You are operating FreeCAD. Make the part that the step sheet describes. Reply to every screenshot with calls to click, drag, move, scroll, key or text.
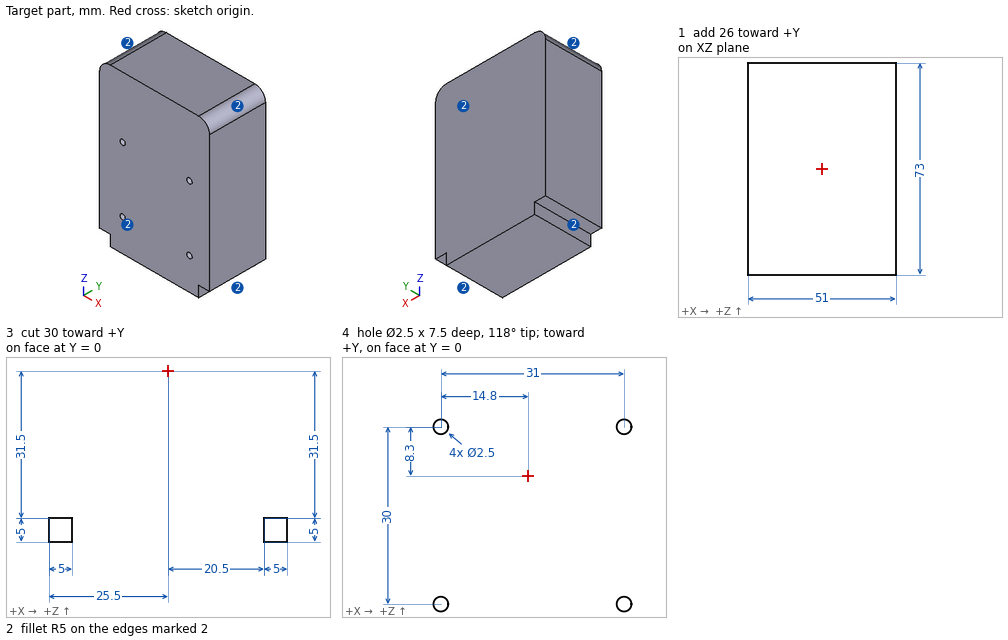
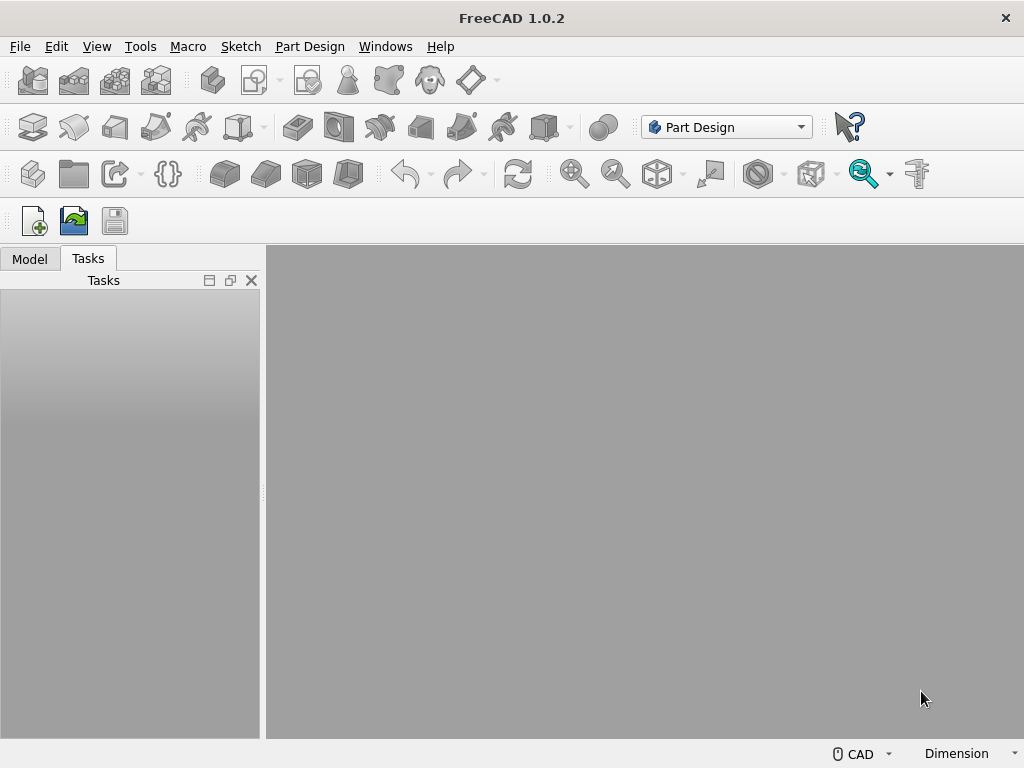
key(ctrl+n)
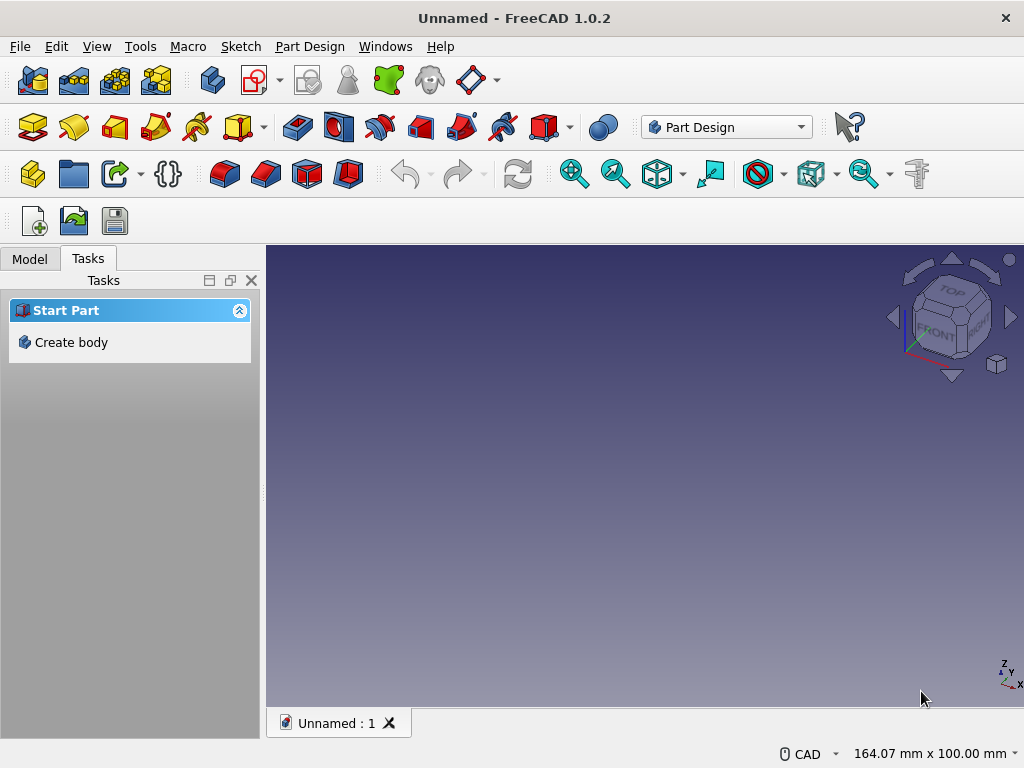
click(254, 80)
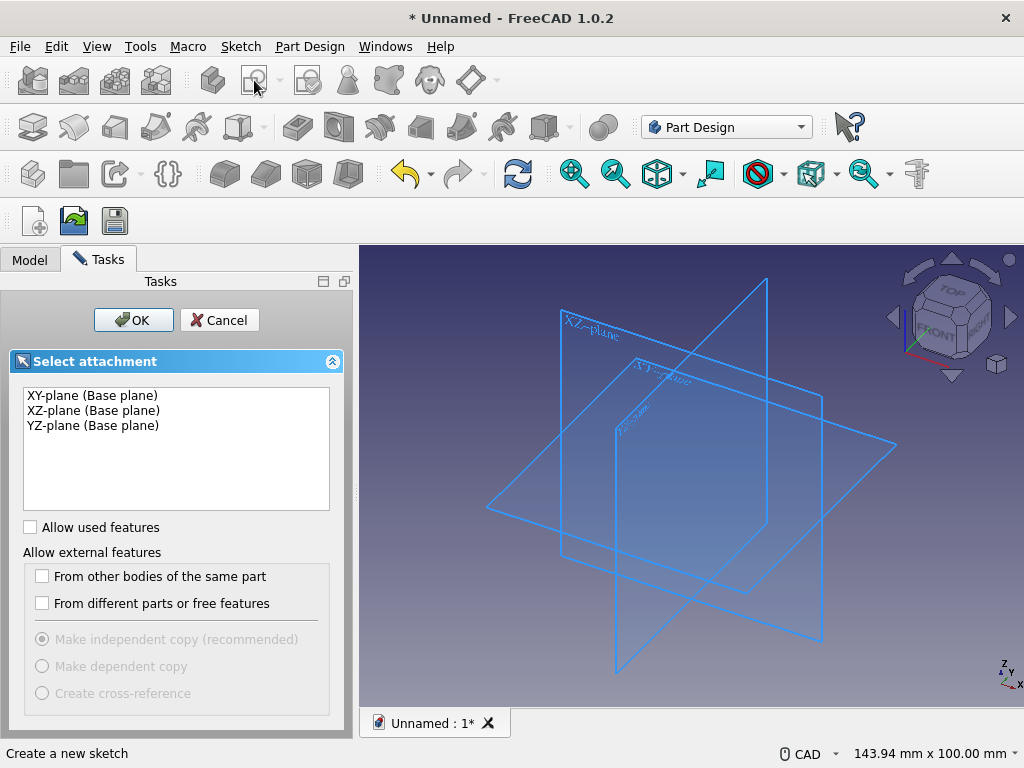
click(84, 410)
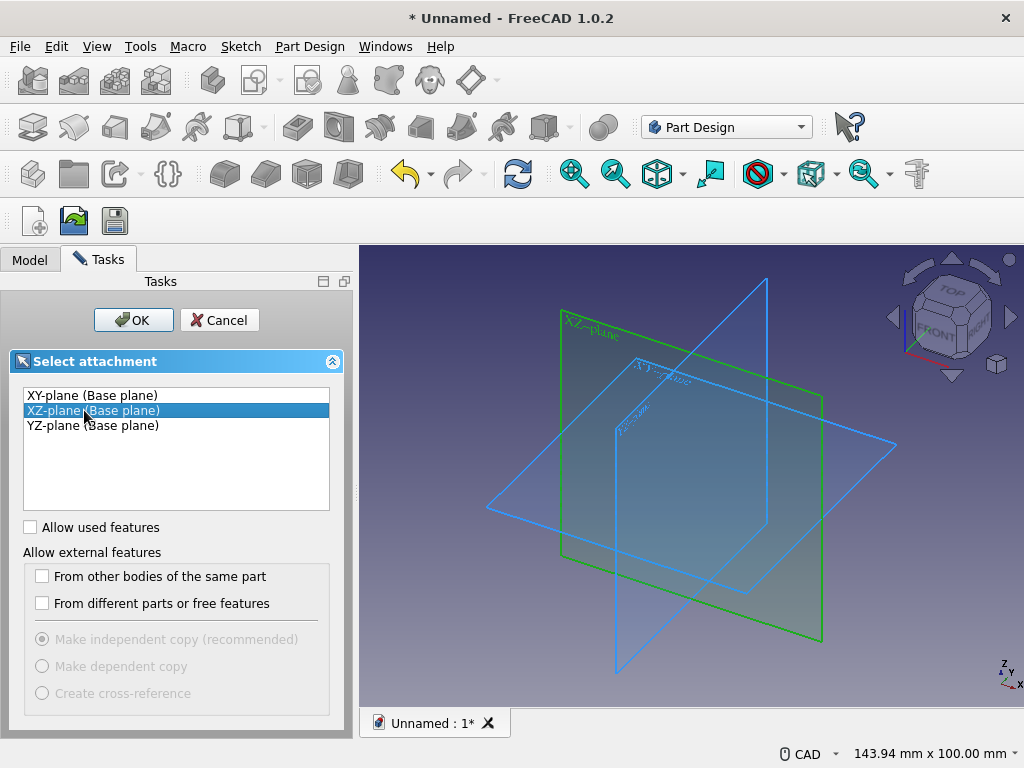
click(134, 320)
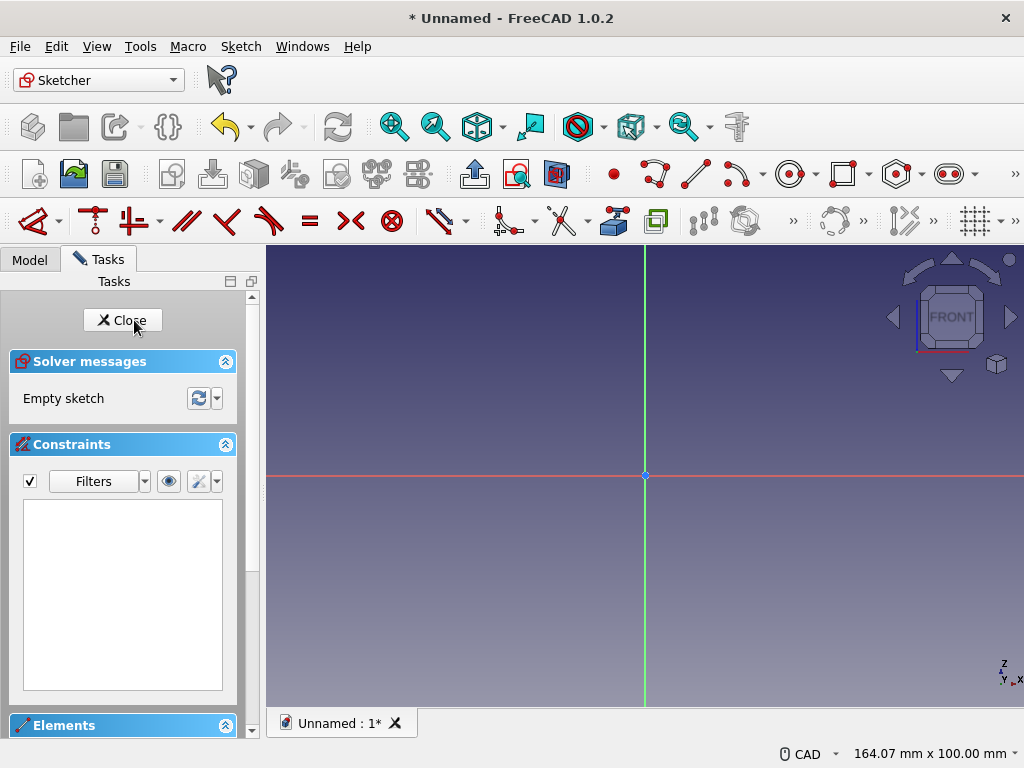
click(868, 174)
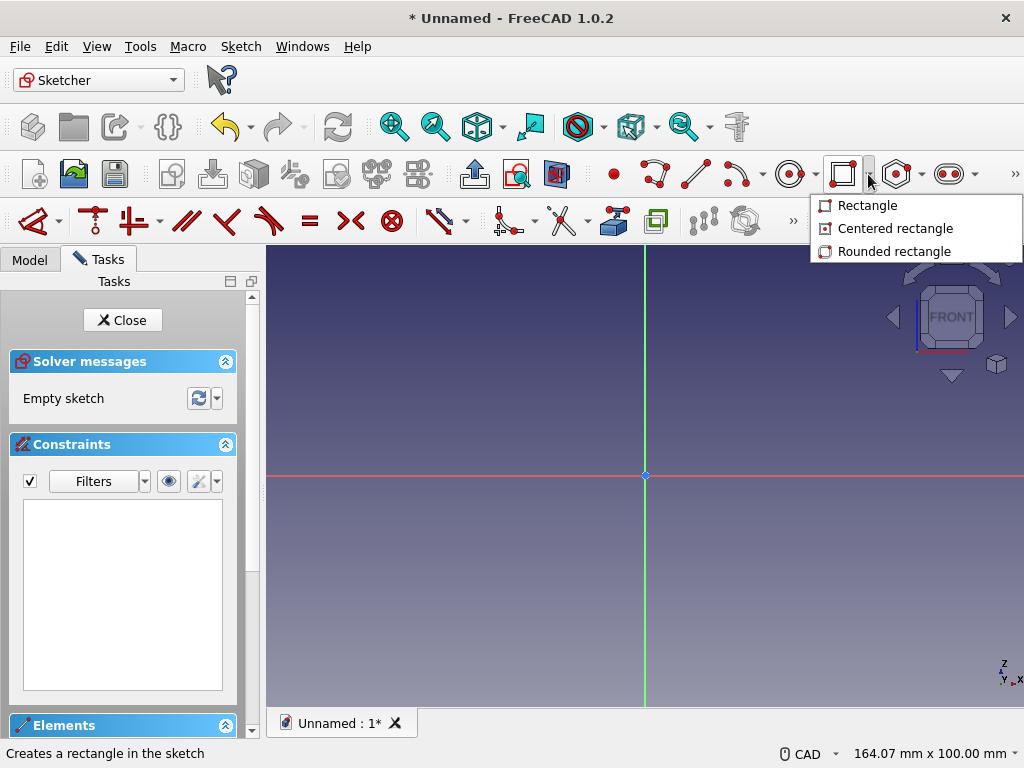
click(916, 228)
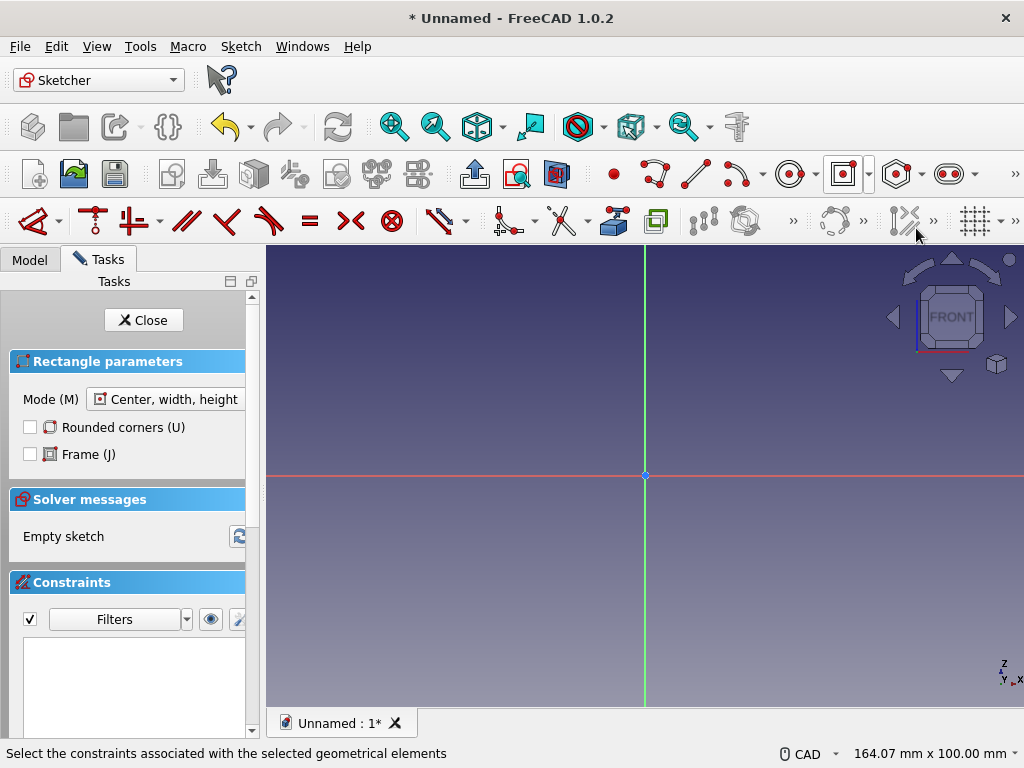
click(645, 476)
click(763, 307)
key(Escape)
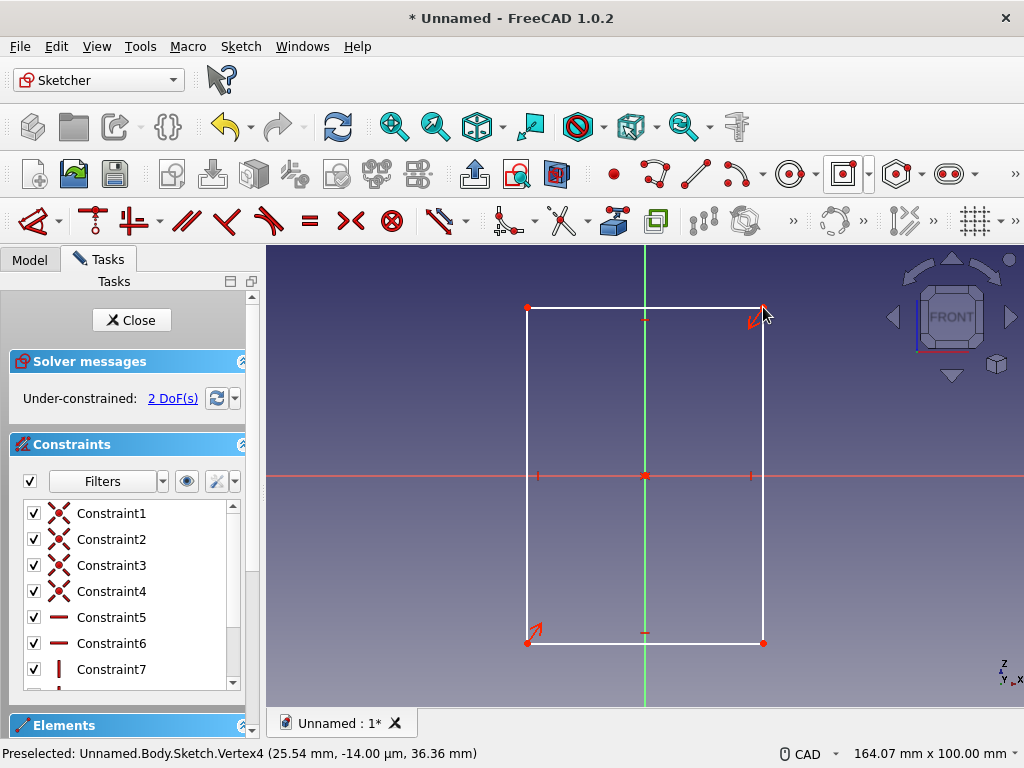
click(598, 644)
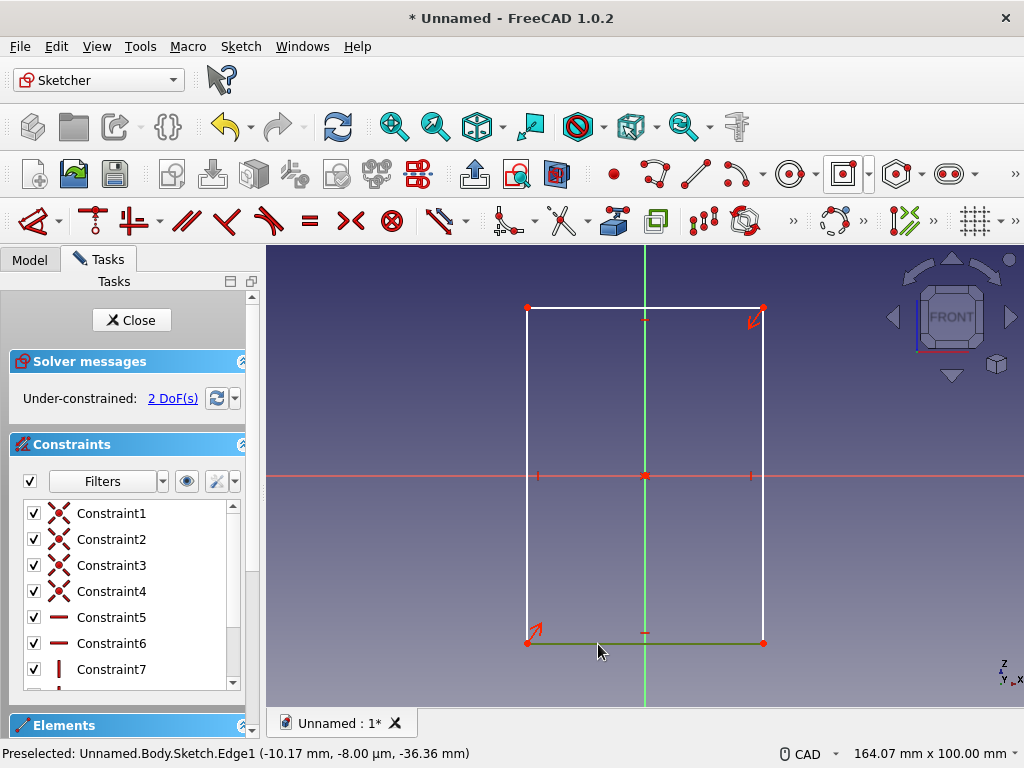
key(l)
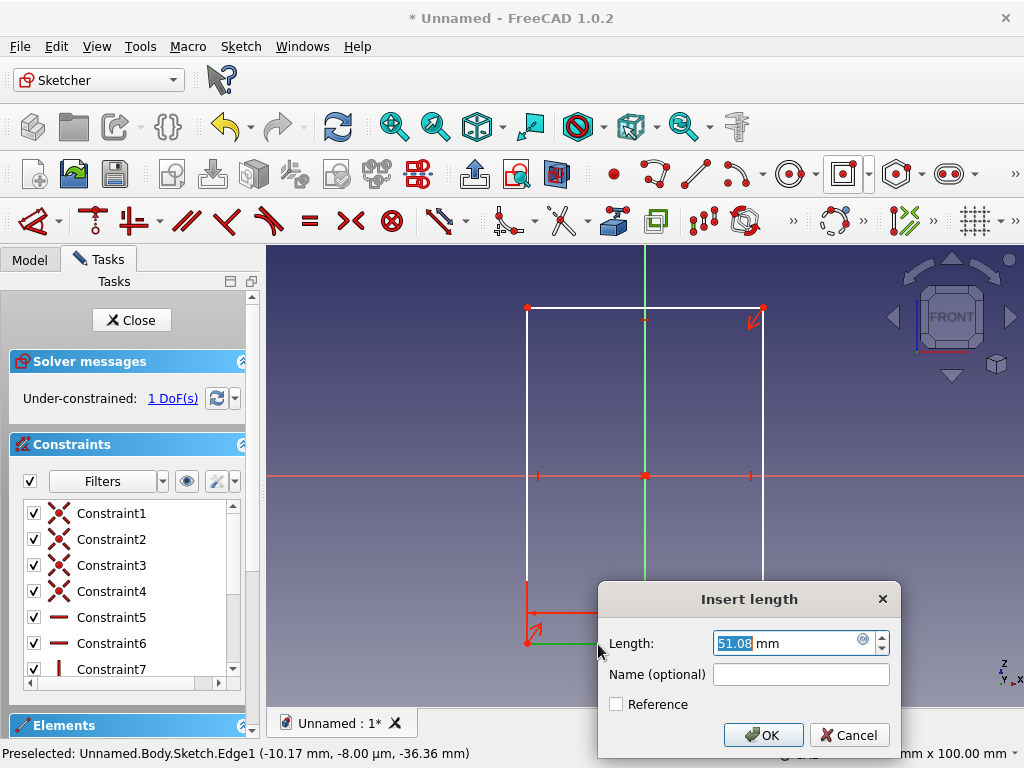
text(51)
key(Return)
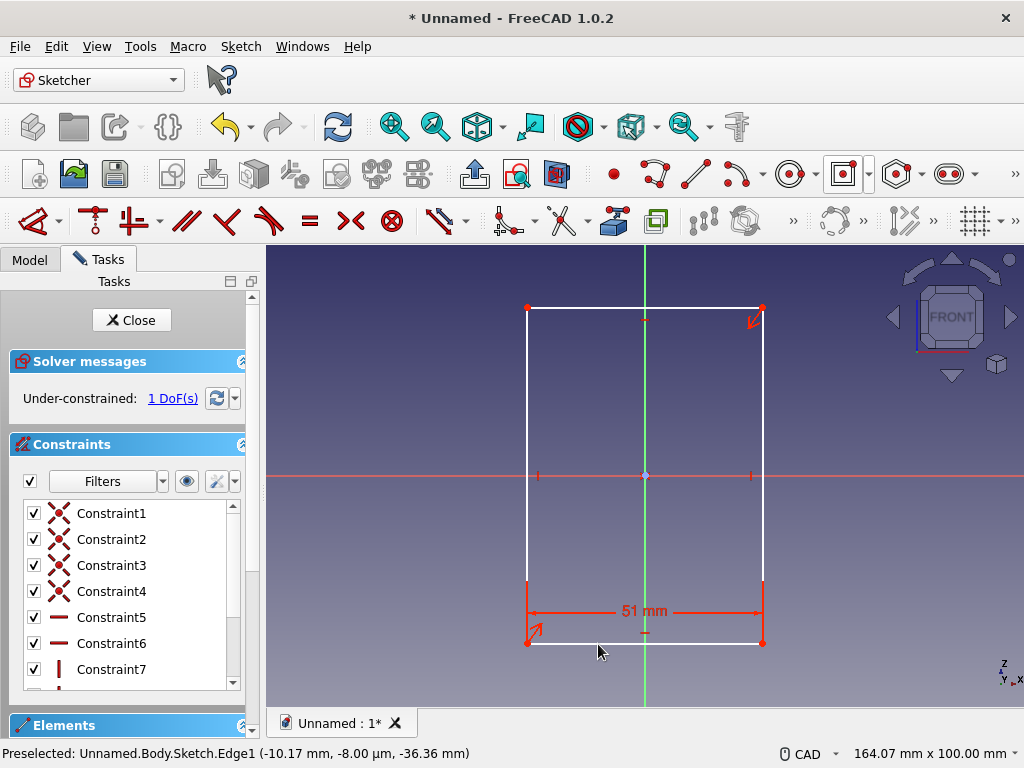
click(763, 543)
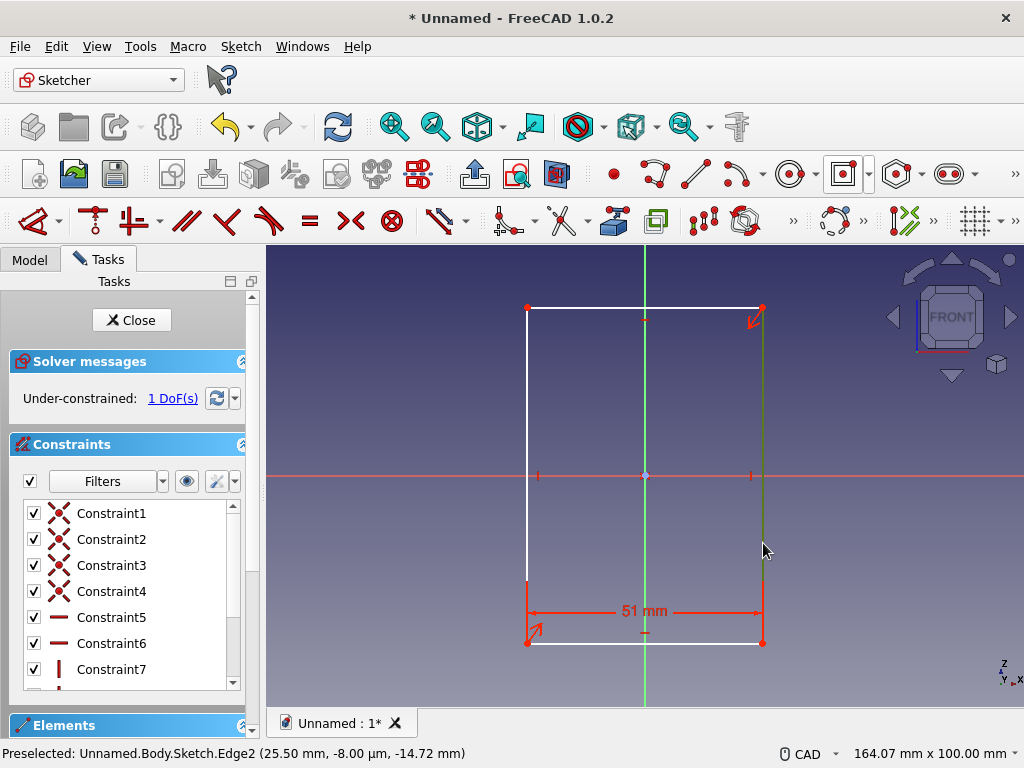
key(i)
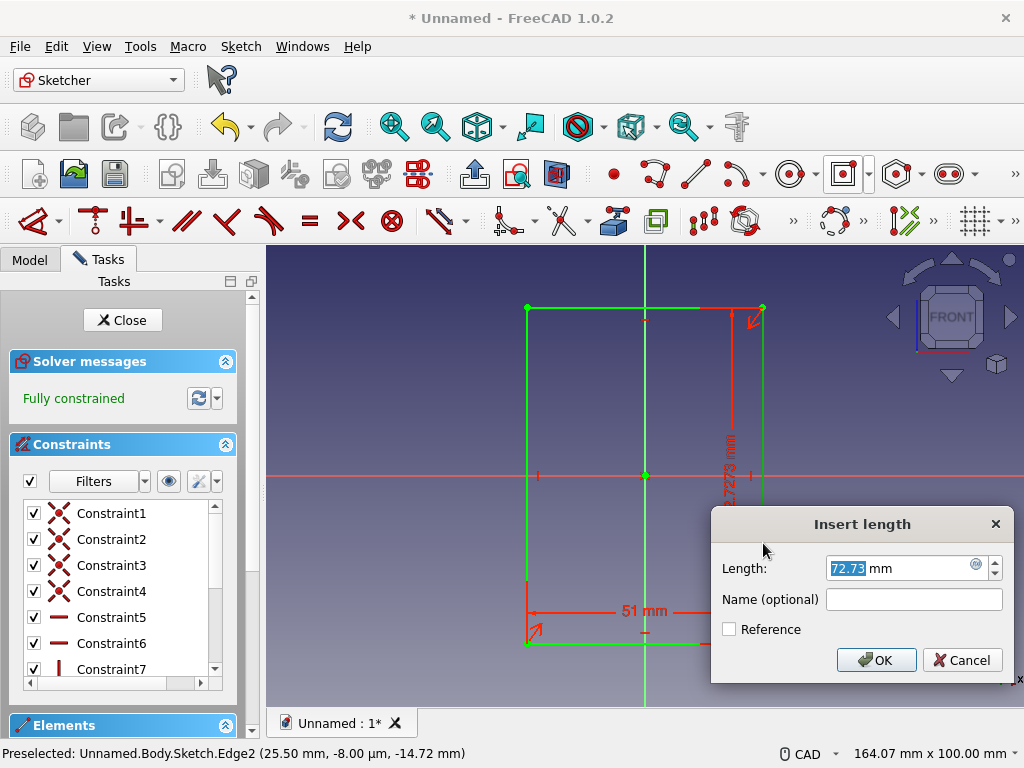
text(73)
key(Return)